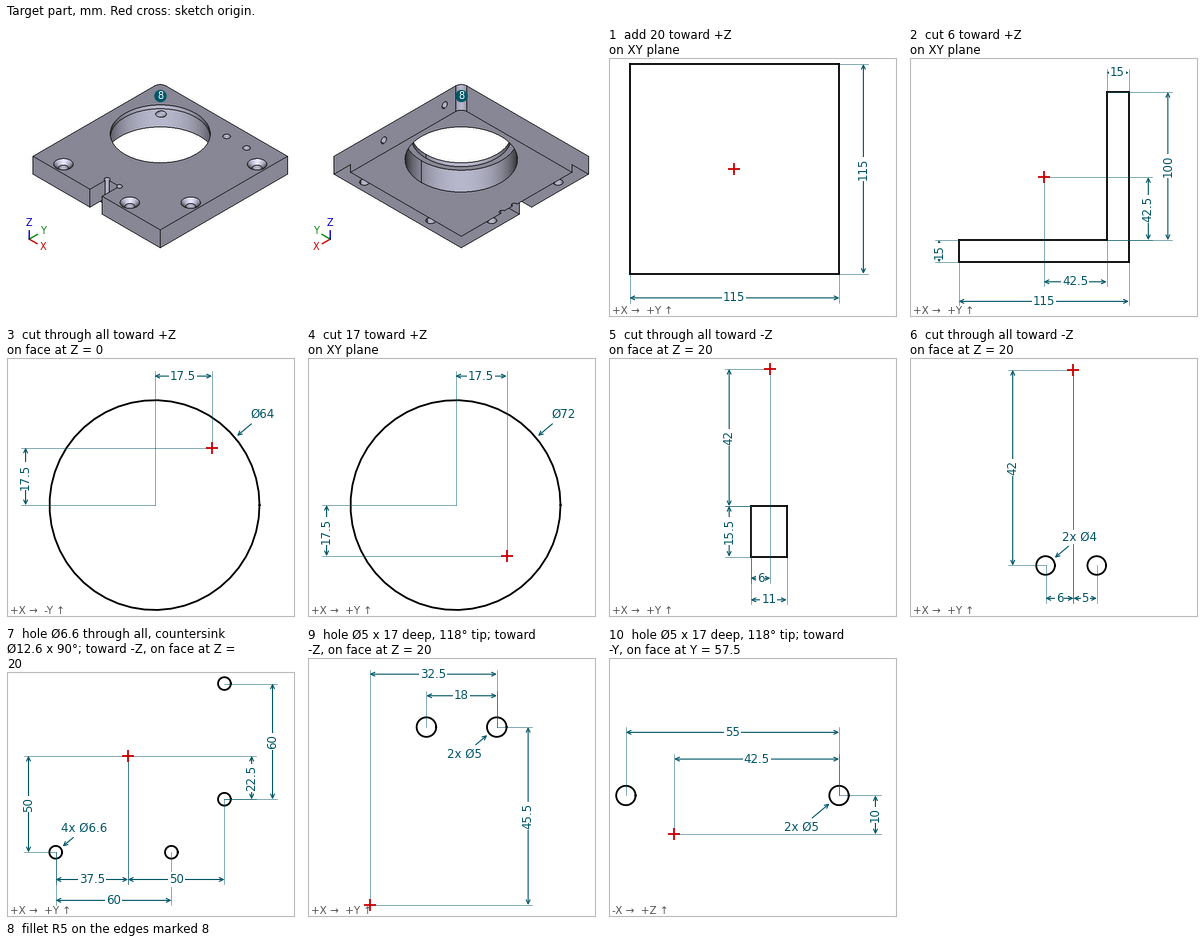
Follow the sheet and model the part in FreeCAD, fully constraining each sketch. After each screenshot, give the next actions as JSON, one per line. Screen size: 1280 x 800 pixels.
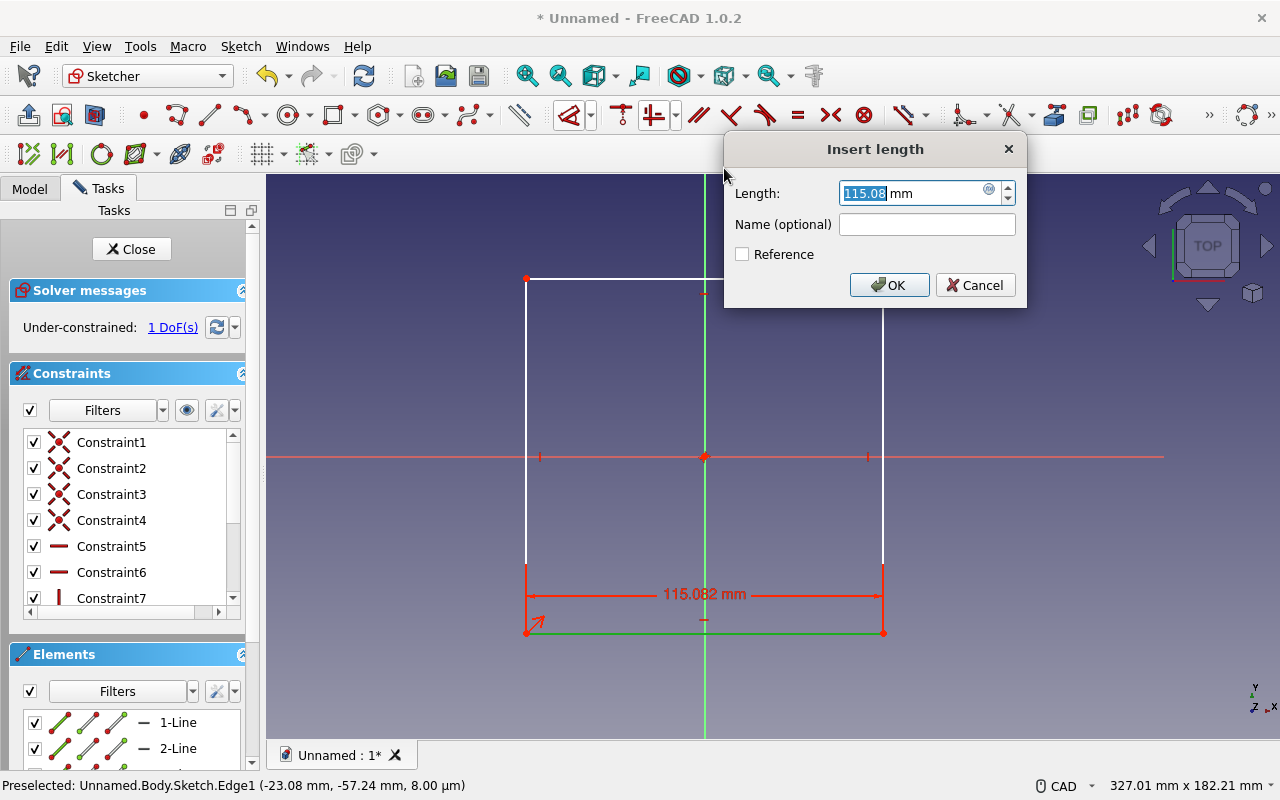
{"action": "type", "text": "115"}
{"action": "key", "text": "Return"}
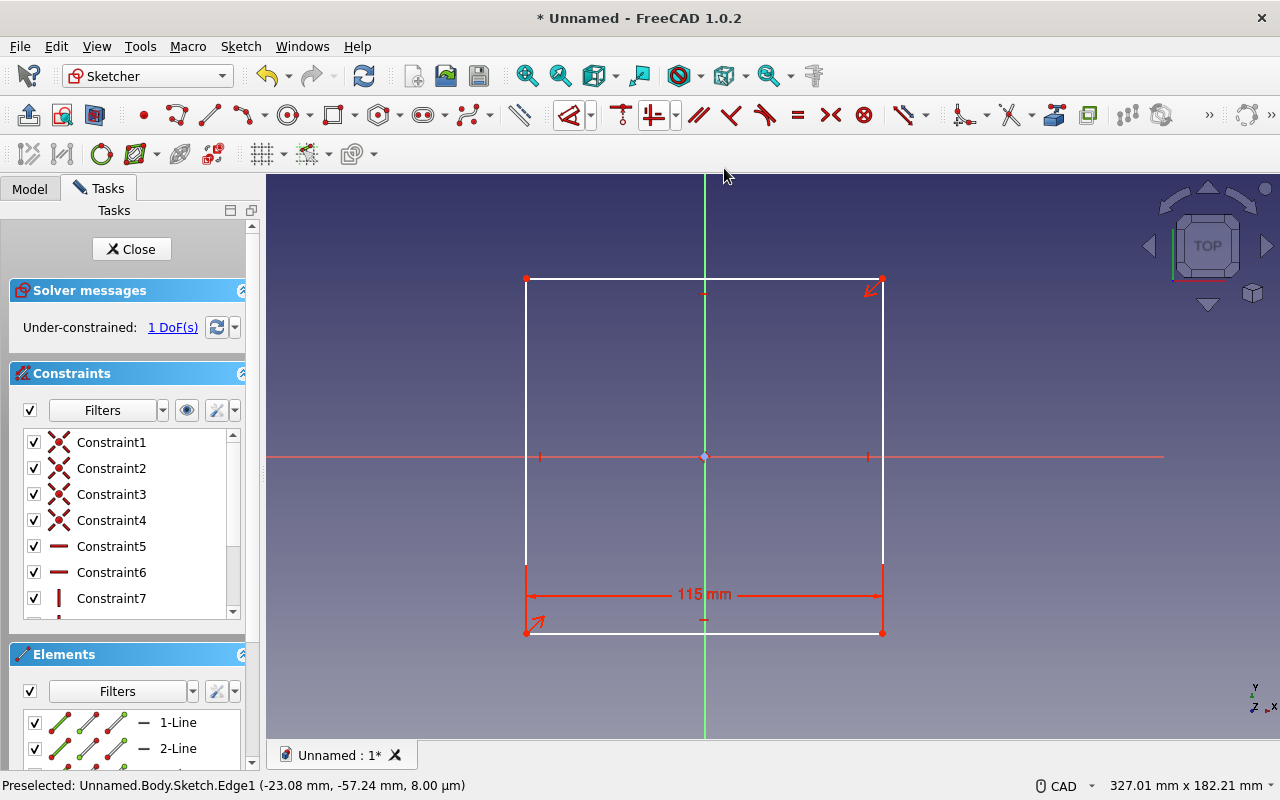
{"action": "left_click", "coordinate": [883, 527]}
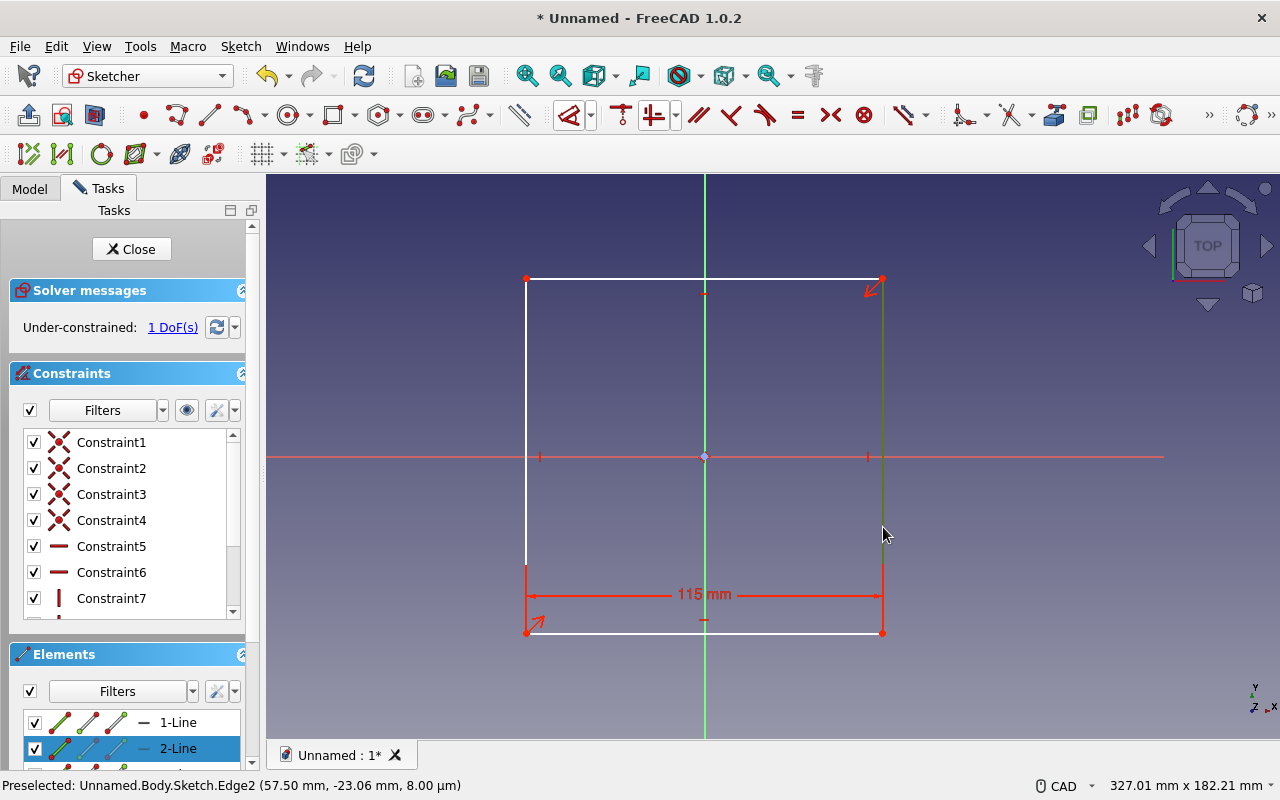
{"action": "left_click", "coordinate": [590, 116]}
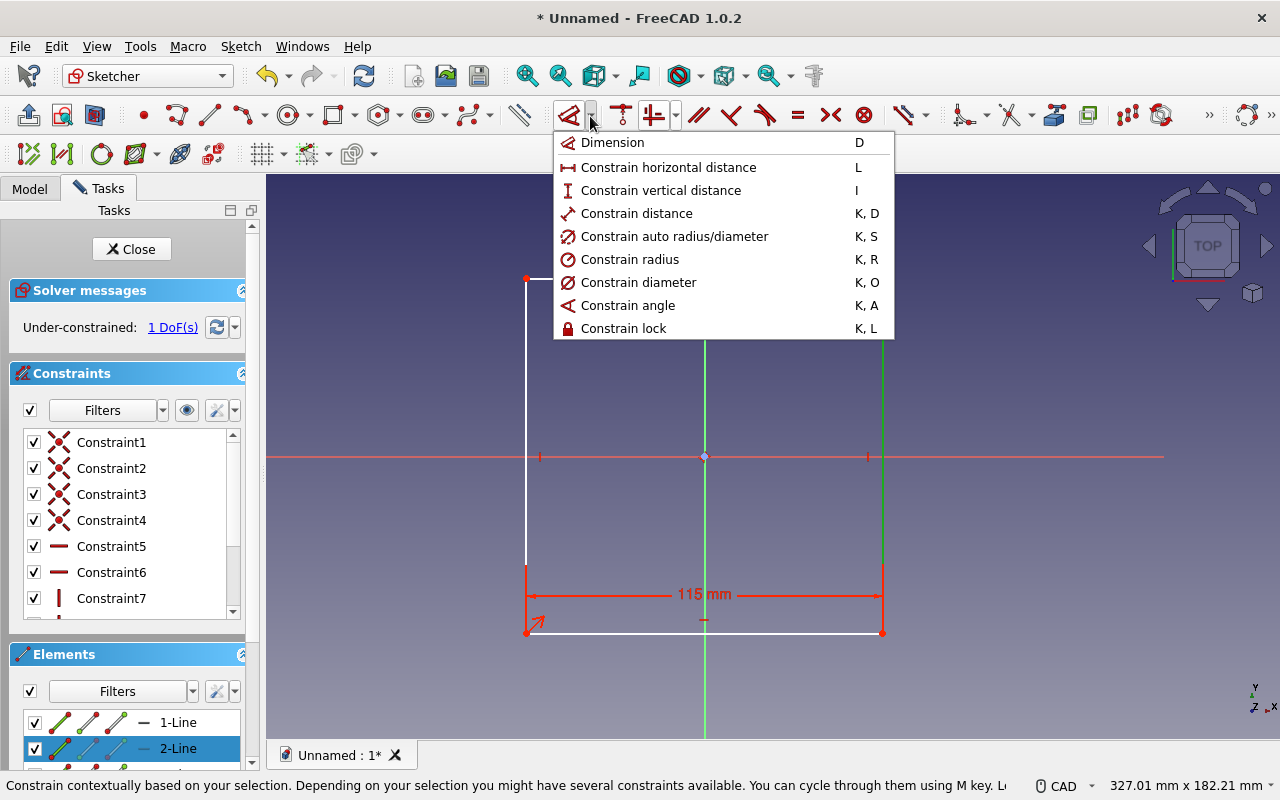
{"action": "left_click", "coordinate": [724, 190]}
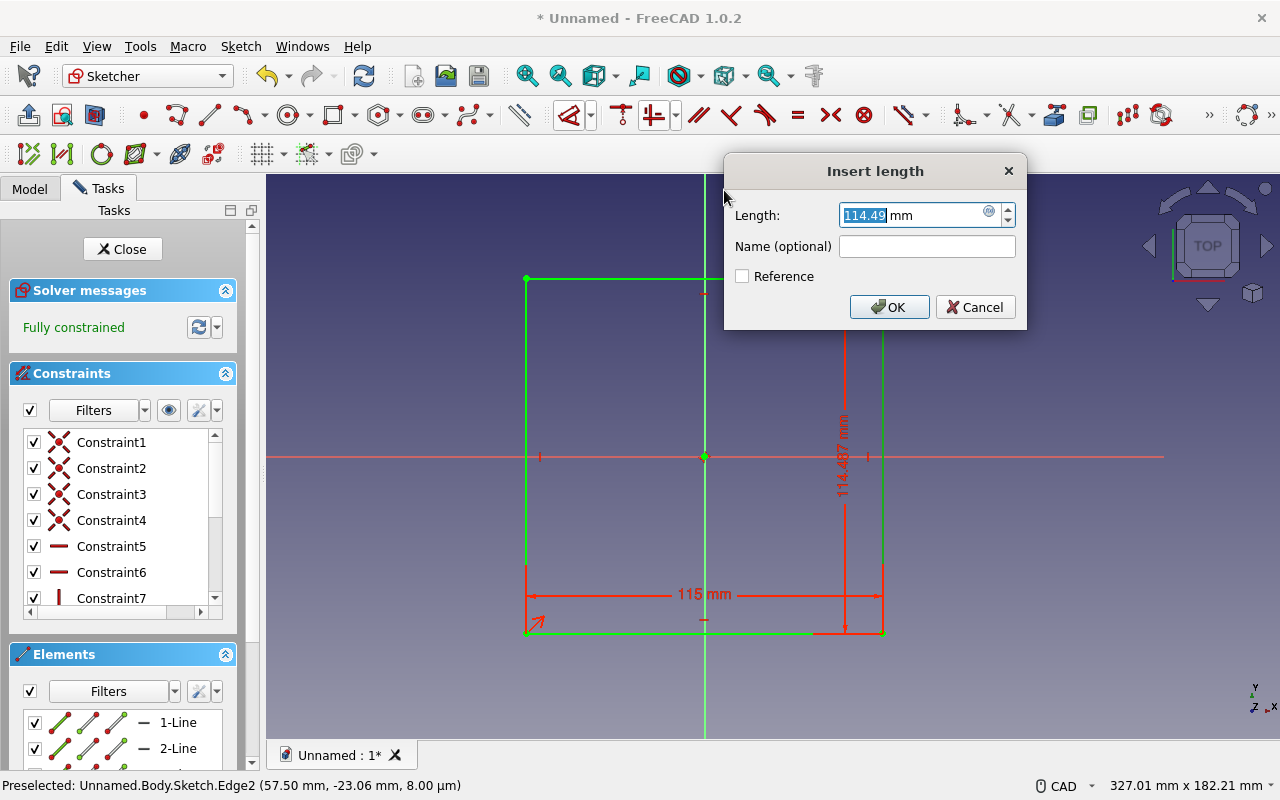
{"action": "type", "text": "115"}
{"action": "key", "text": "Return"}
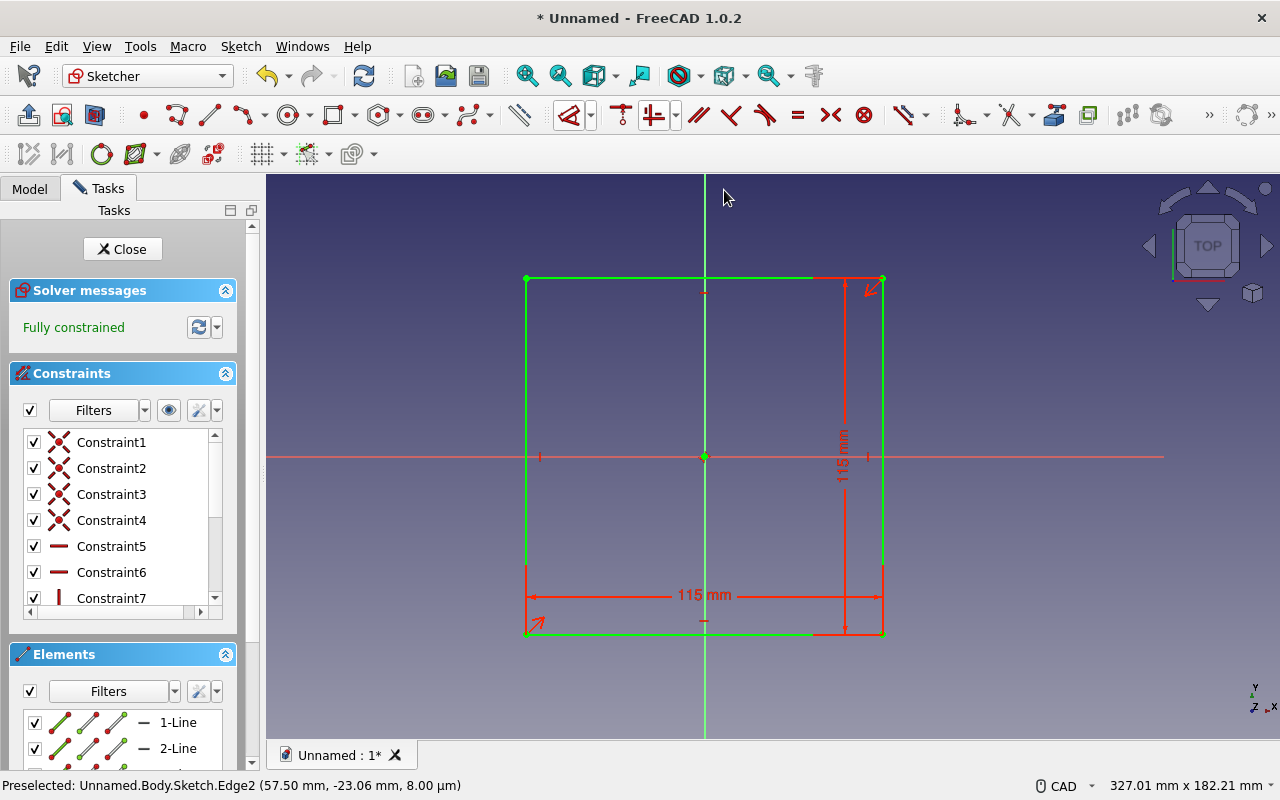
{"action": "left_click", "coordinate": [123, 249]}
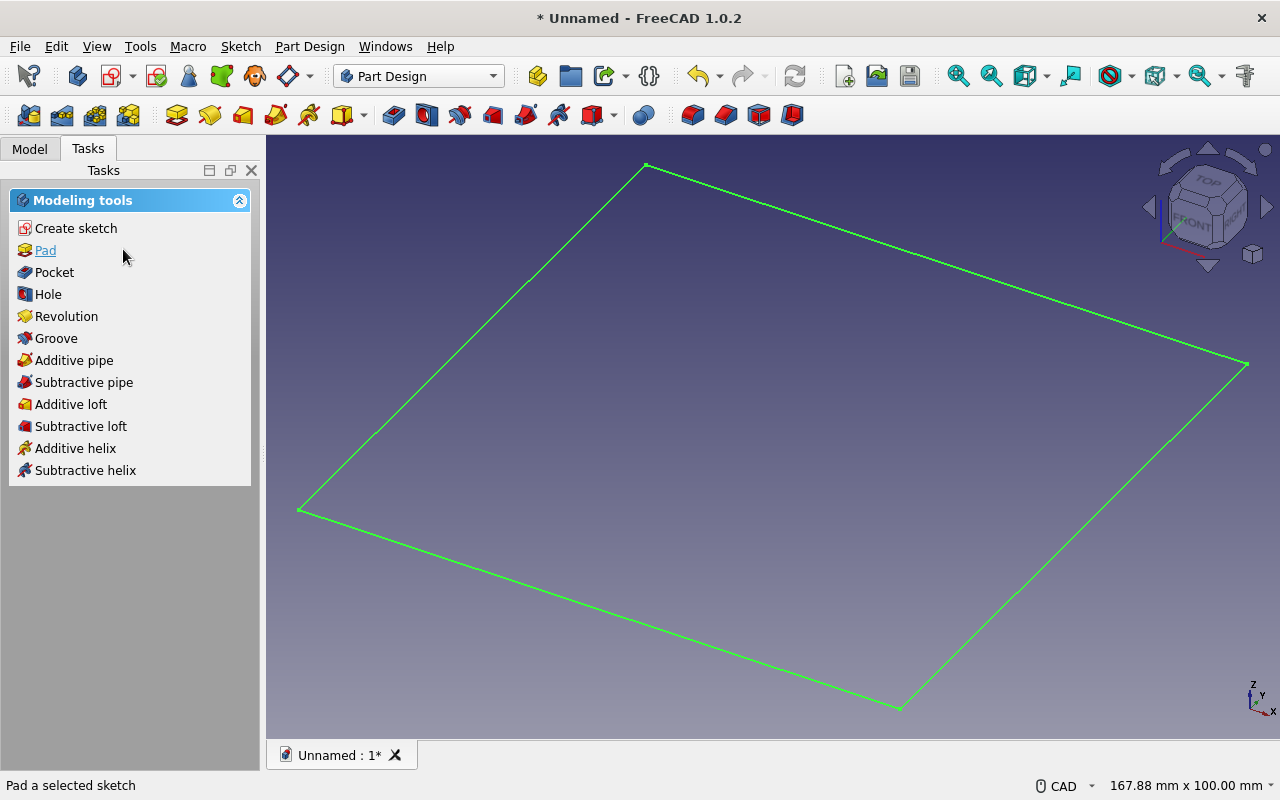
{"action": "left_click", "coordinate": [177, 116]}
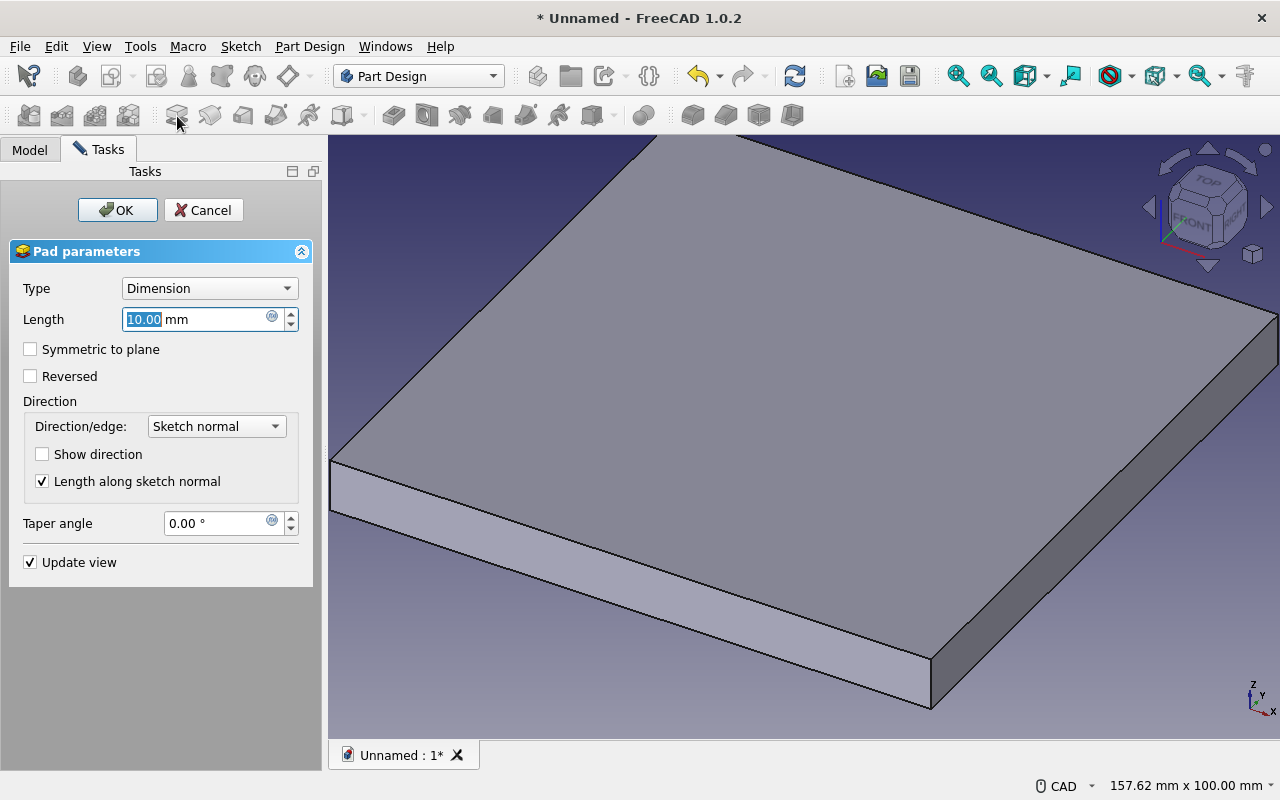
{"action": "type", "text": "20"}
{"action": "key", "text": "Tab"}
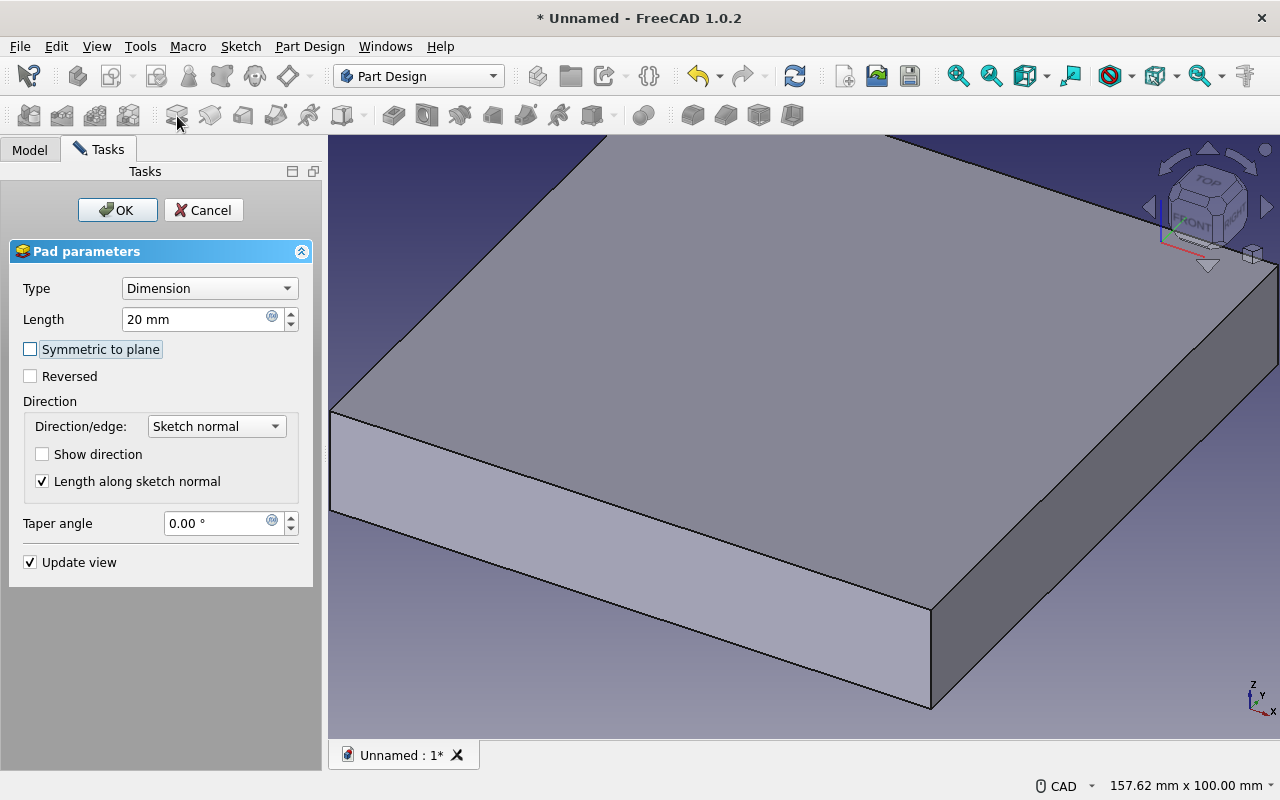
{"action": "left_click", "coordinate": [118, 210]}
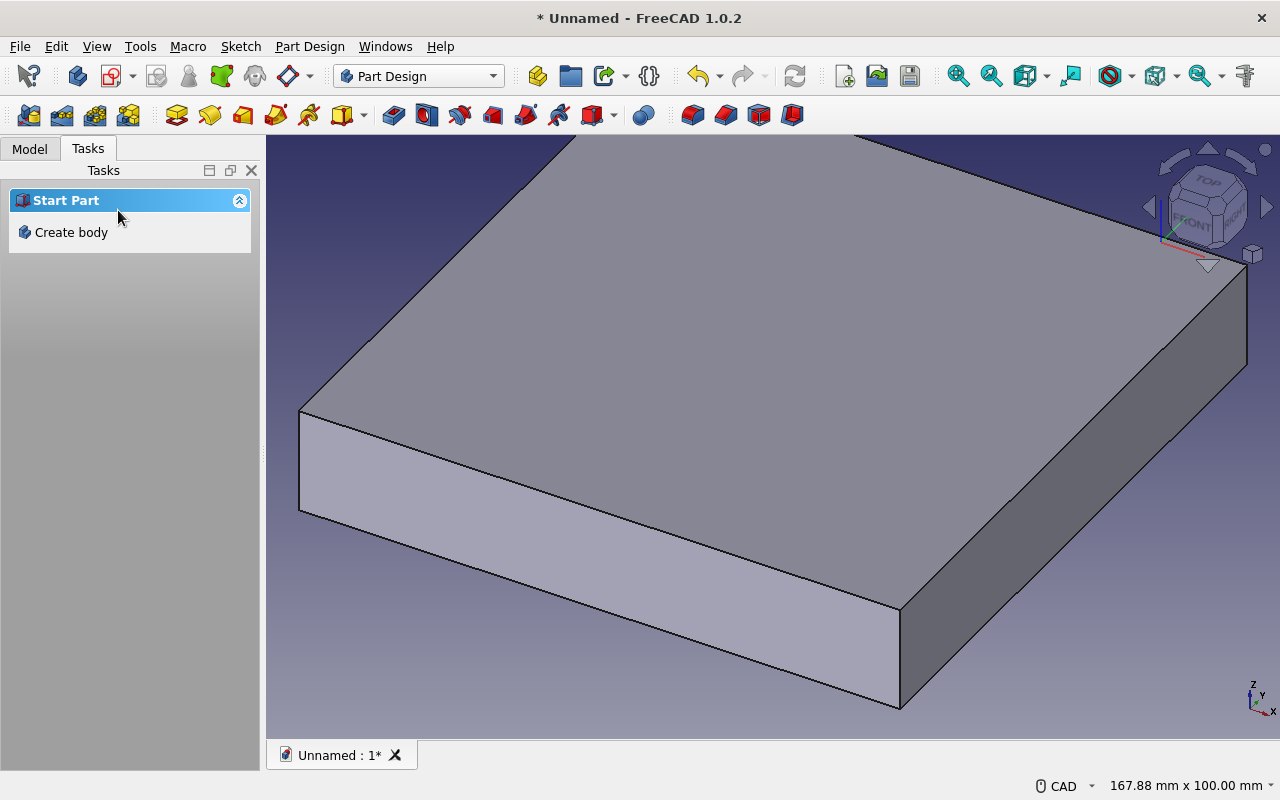
{"action": "left_click", "coordinate": [959, 76]}